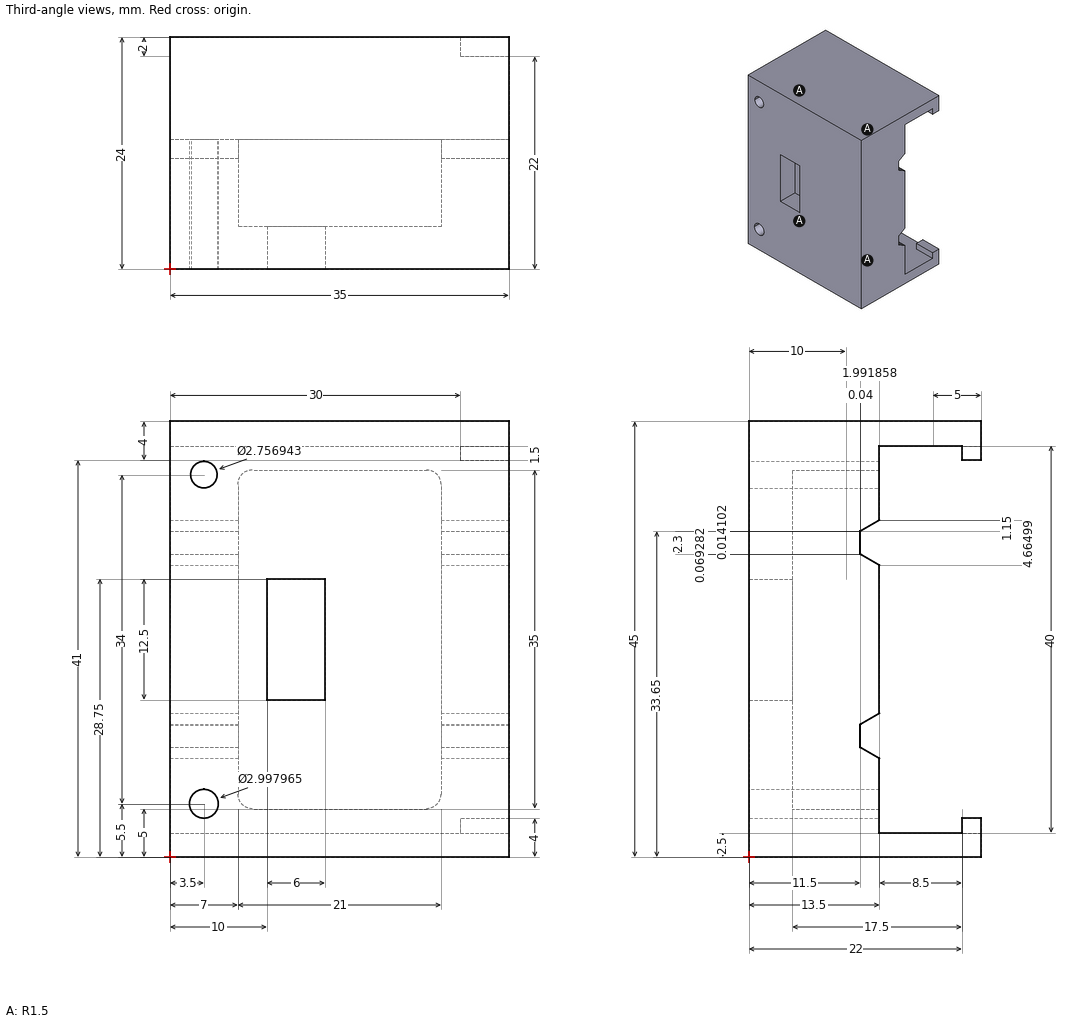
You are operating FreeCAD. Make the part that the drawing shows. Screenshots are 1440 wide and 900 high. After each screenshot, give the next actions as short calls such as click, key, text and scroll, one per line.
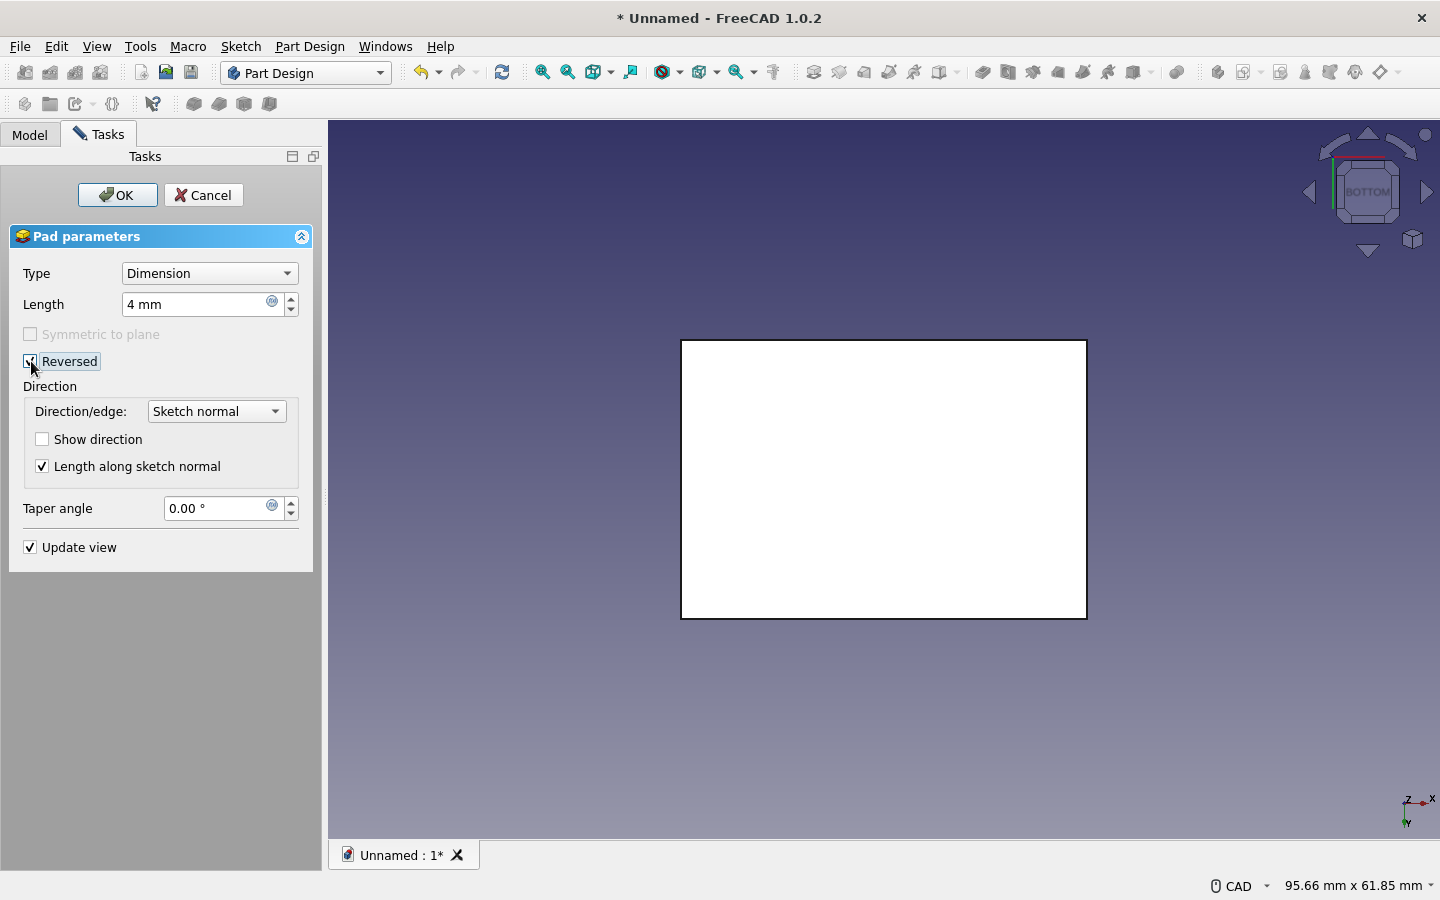
click(118, 195)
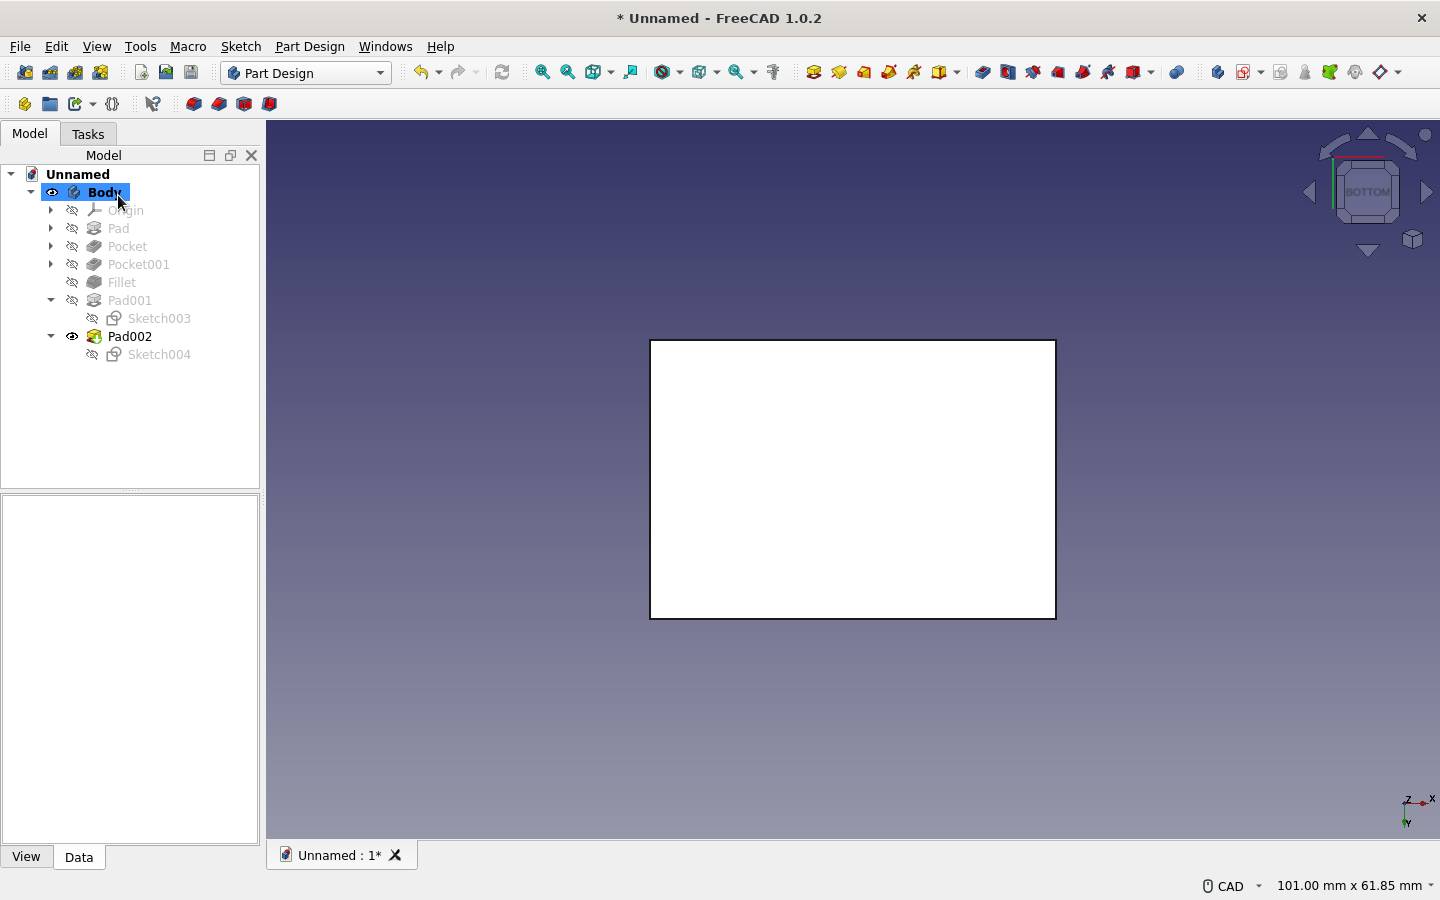
click(543, 72)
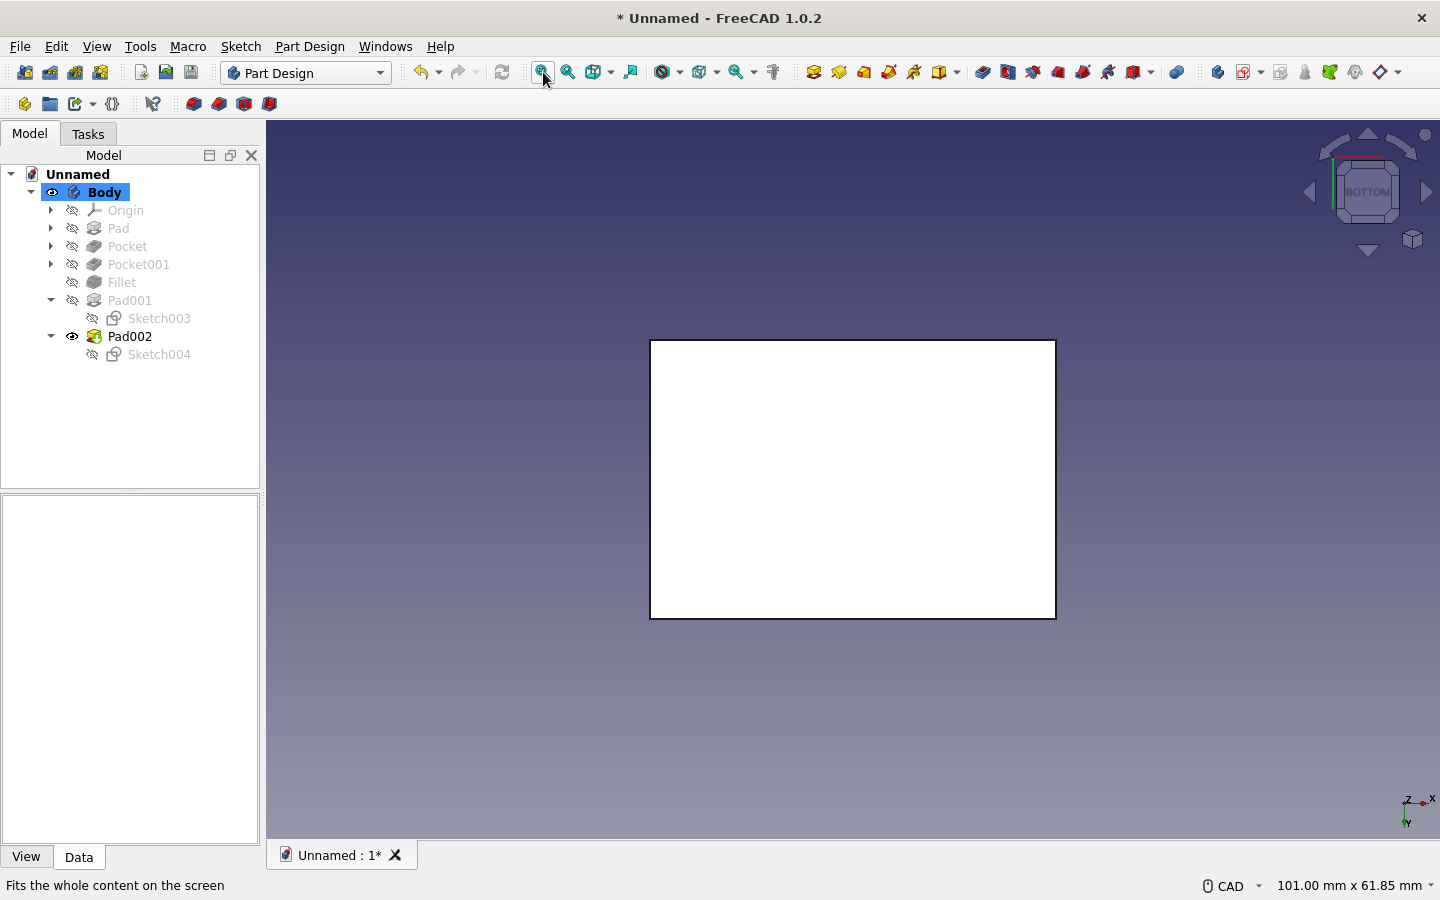
key(4)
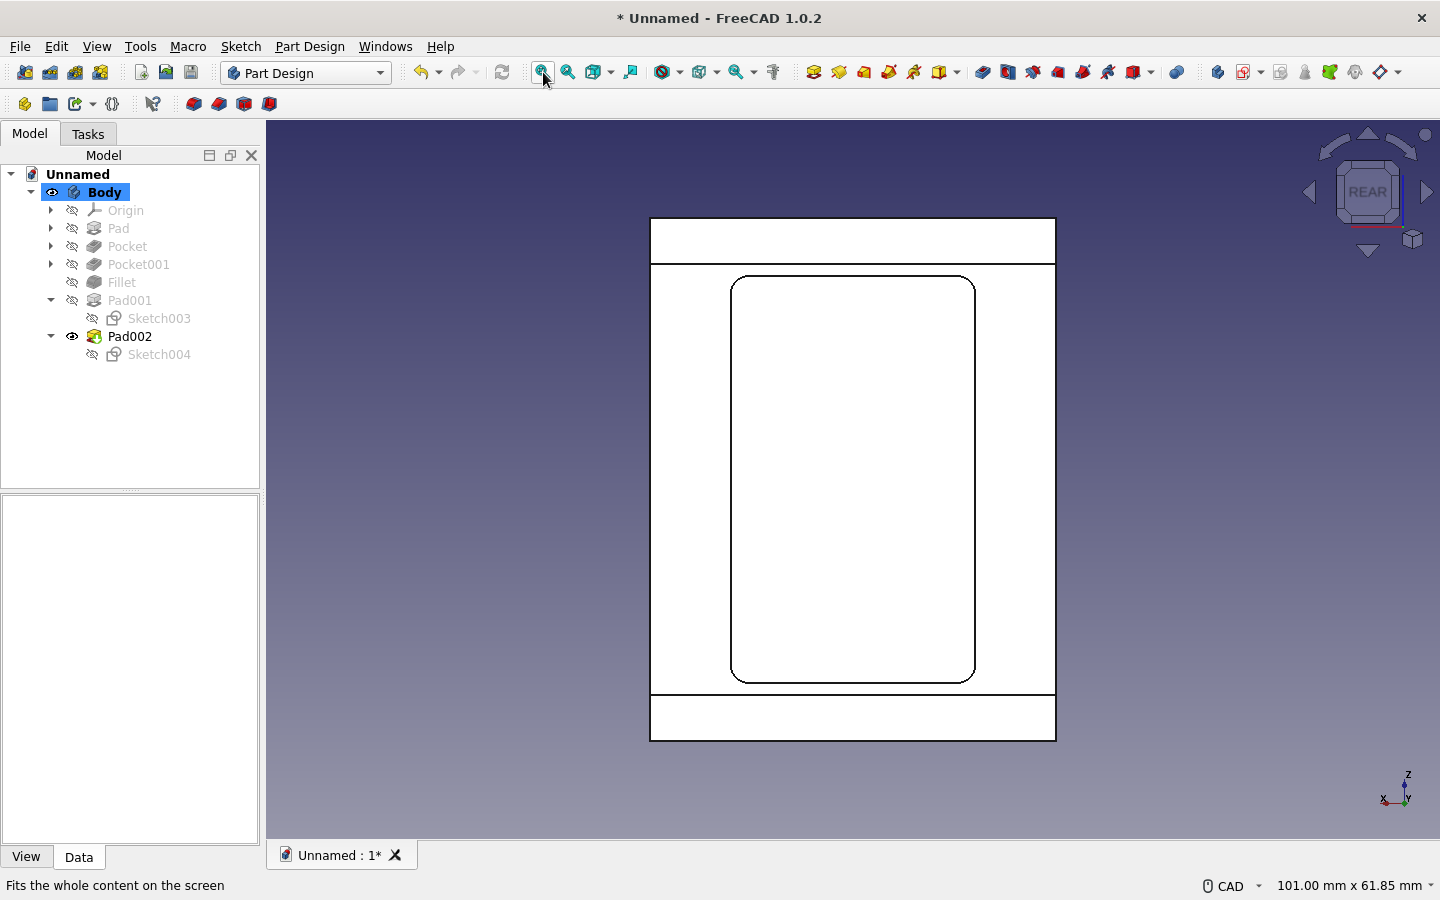
click(679, 279)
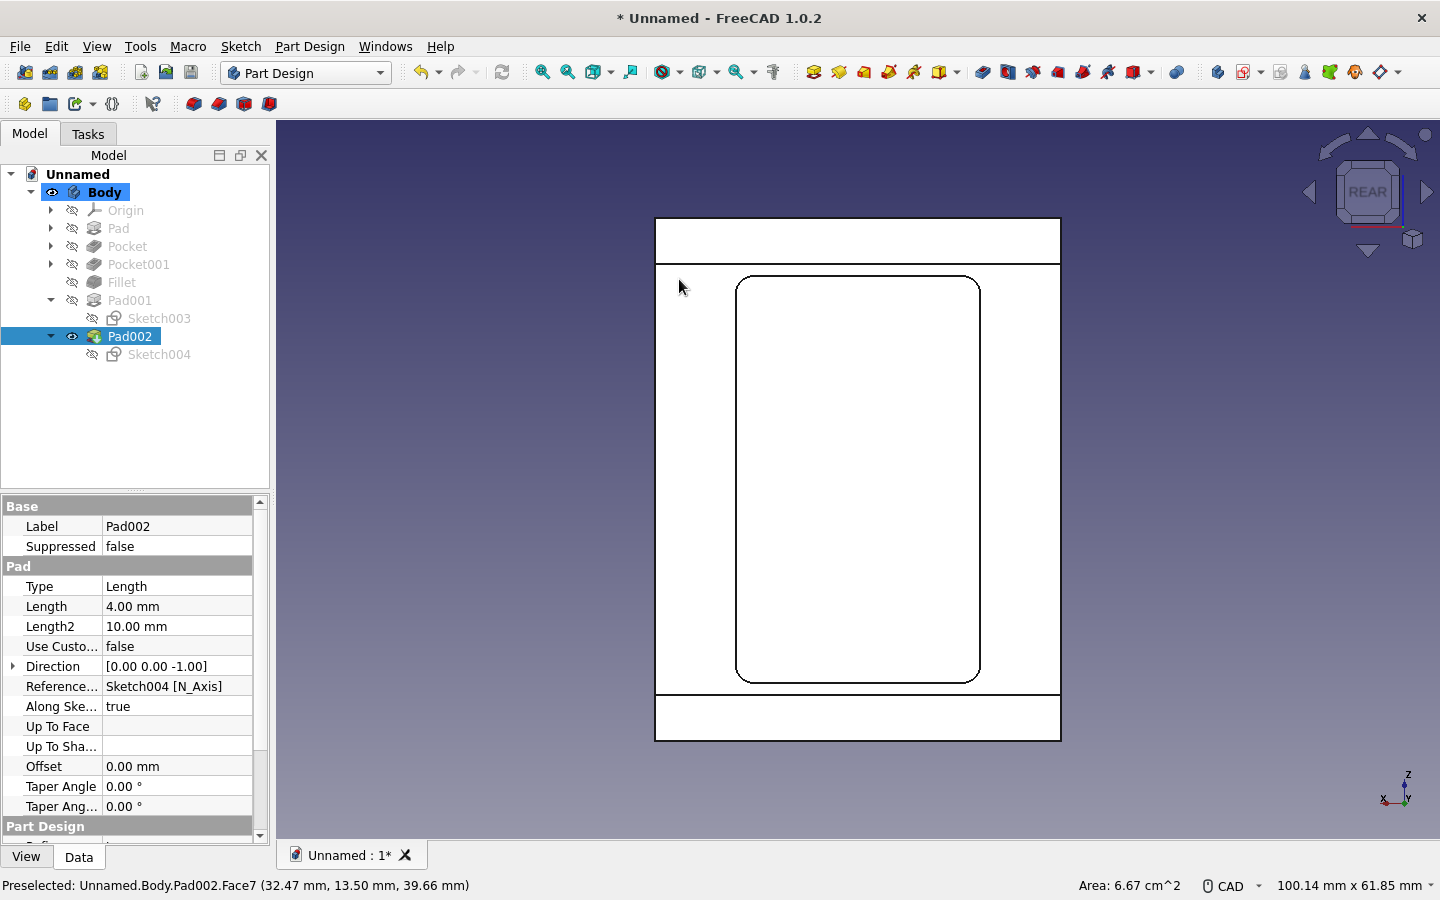
click(1242, 72)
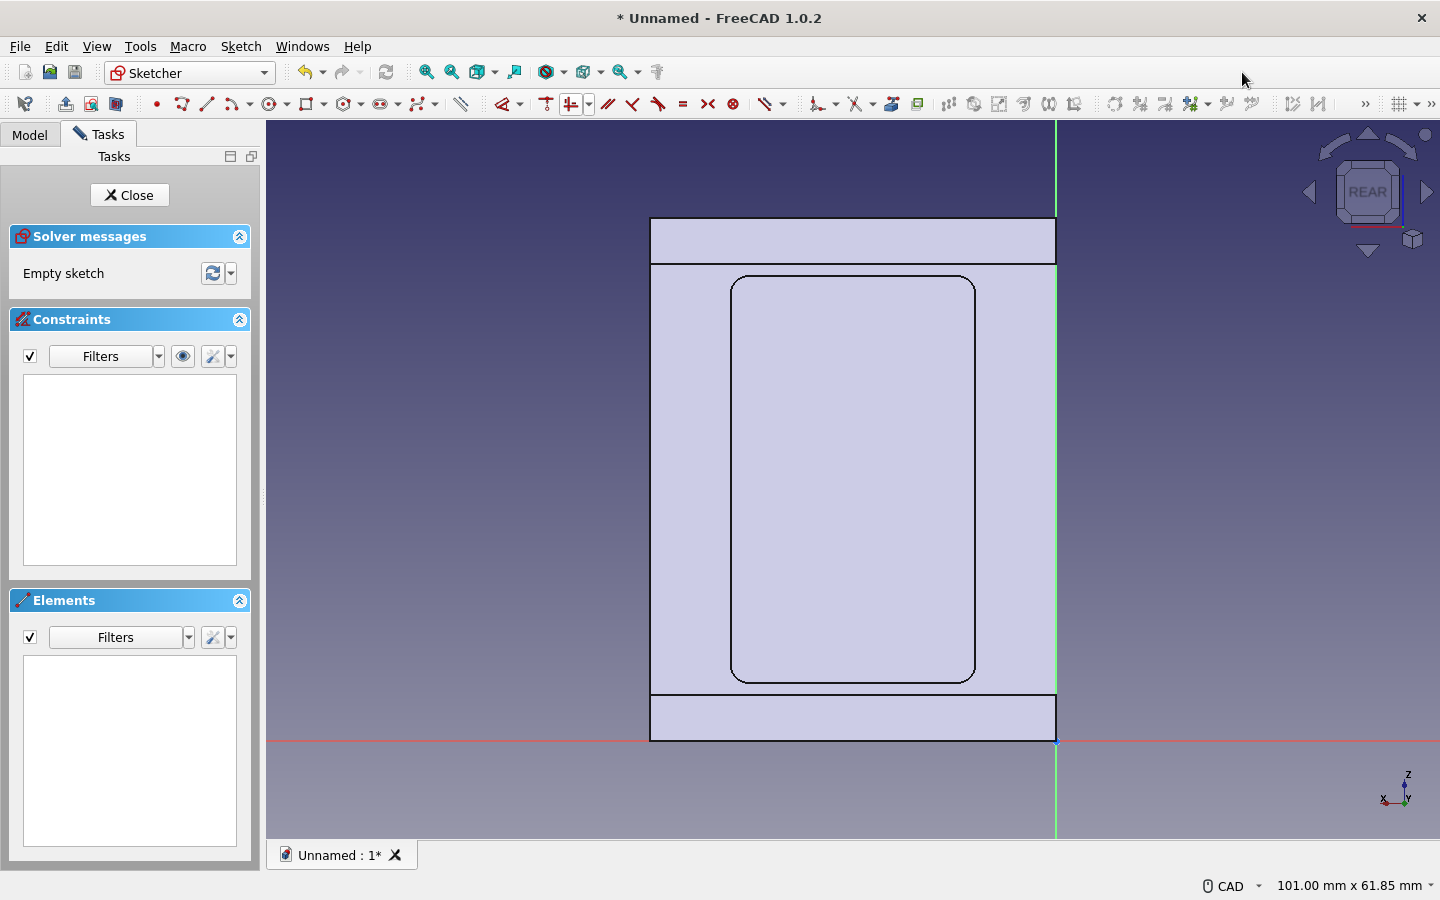
key(q)
key(s)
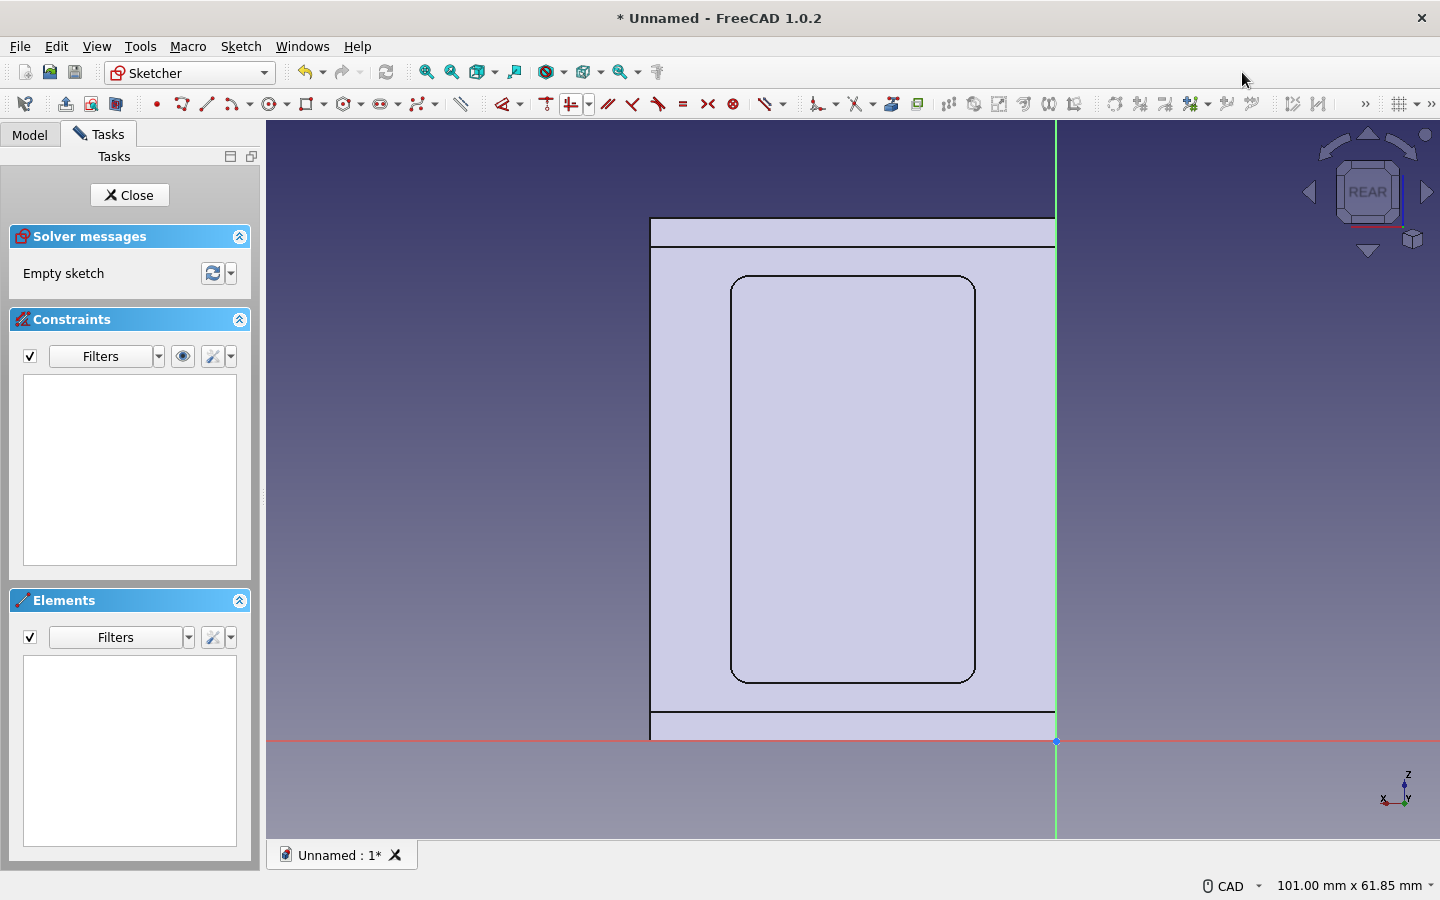
click(268, 104)